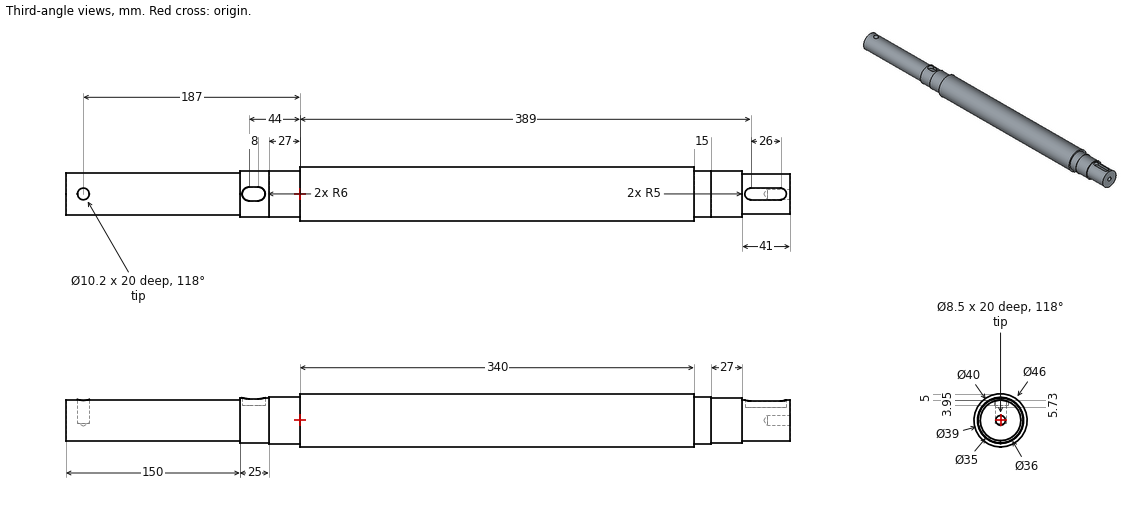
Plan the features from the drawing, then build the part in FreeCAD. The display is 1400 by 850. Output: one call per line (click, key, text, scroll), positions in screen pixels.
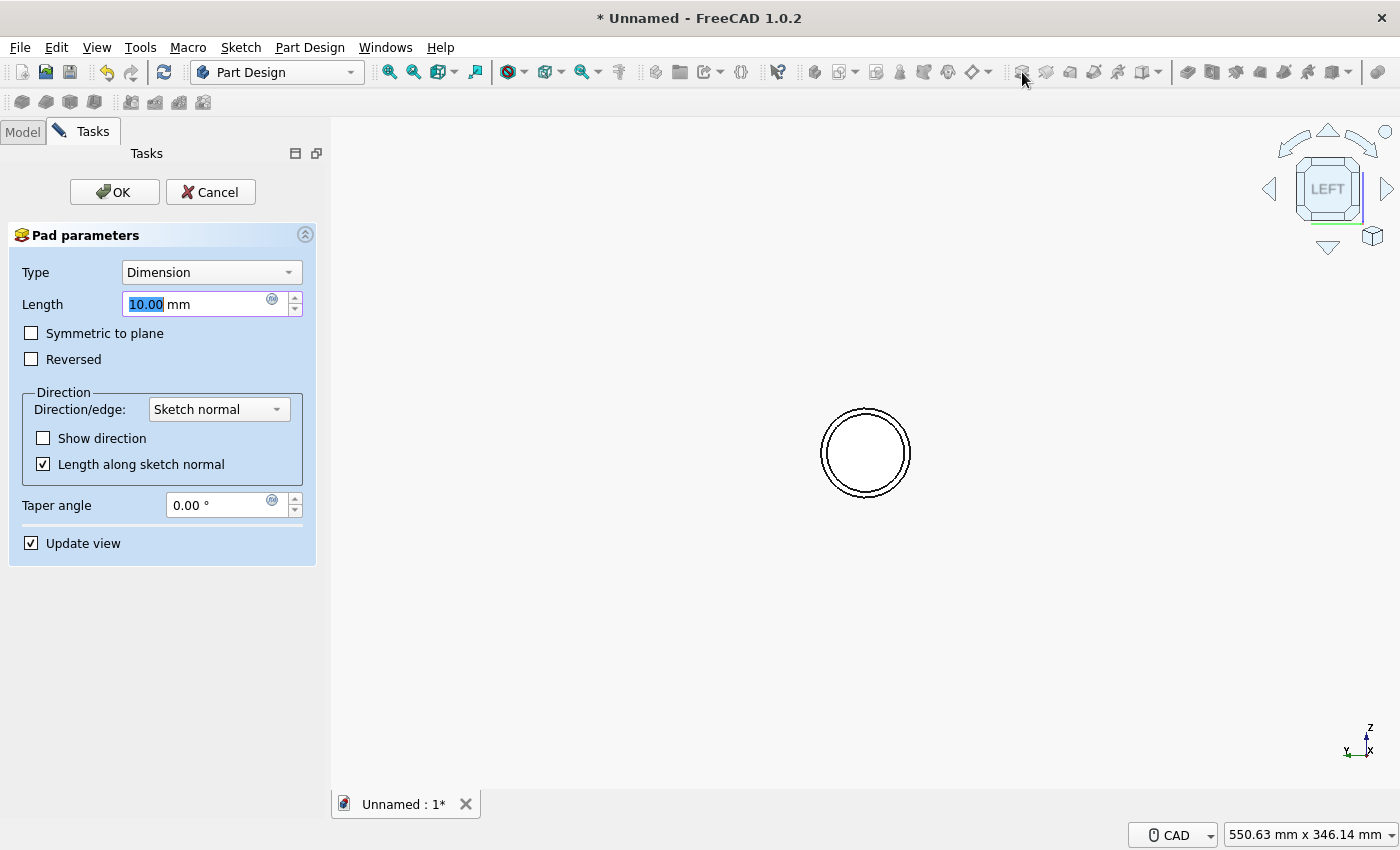
text(27)
key(Tab)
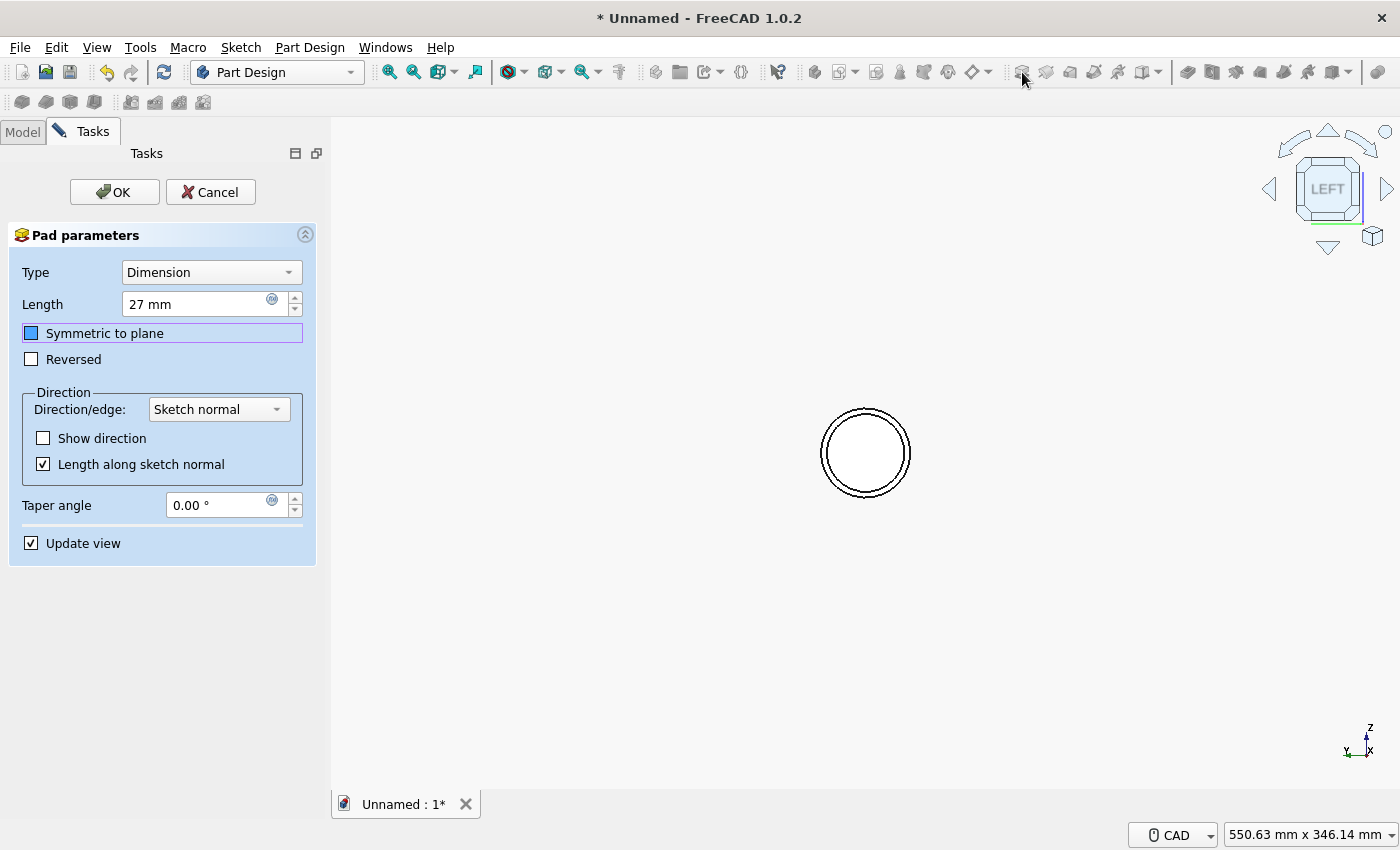
click(115, 192)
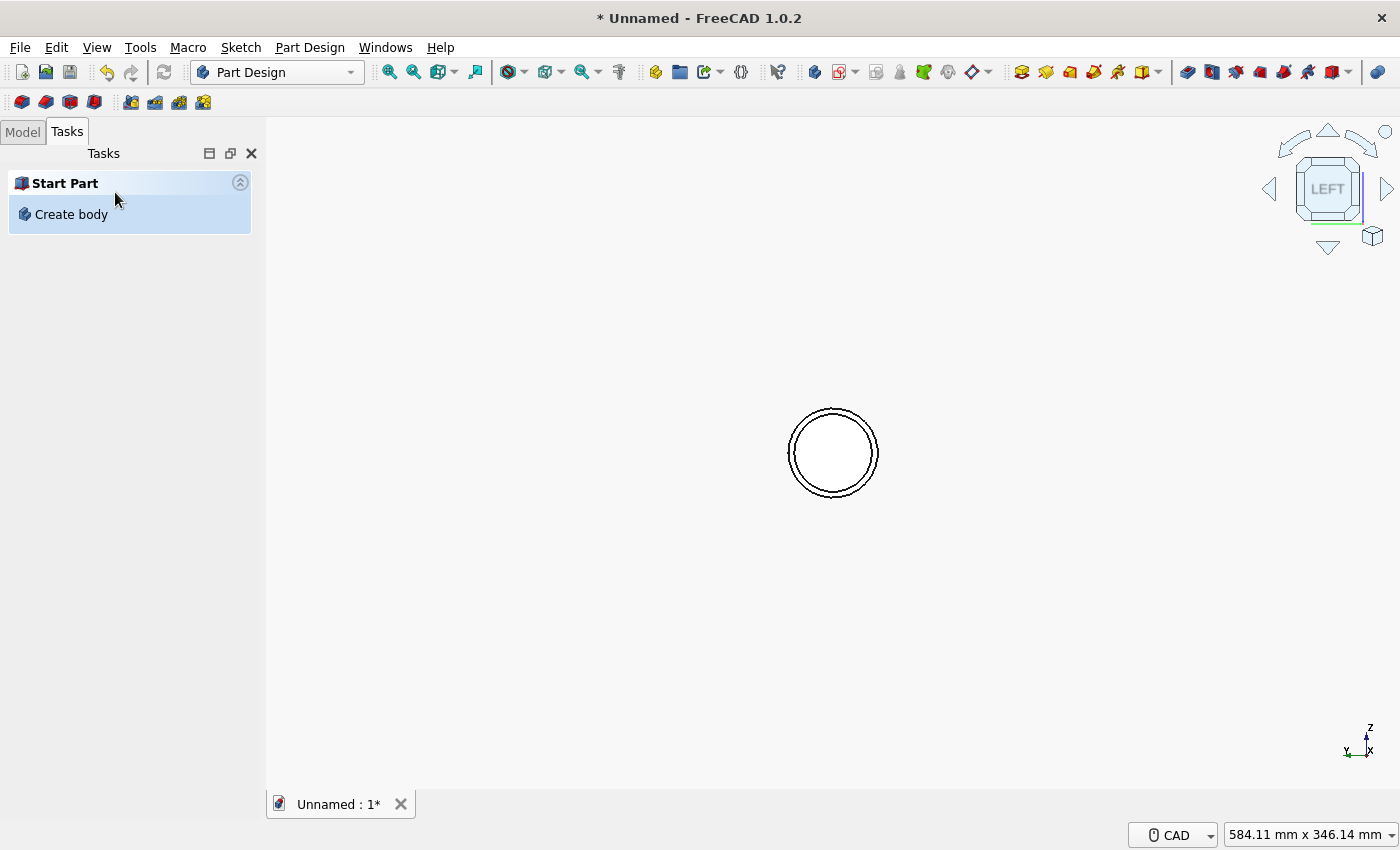
click(390, 72)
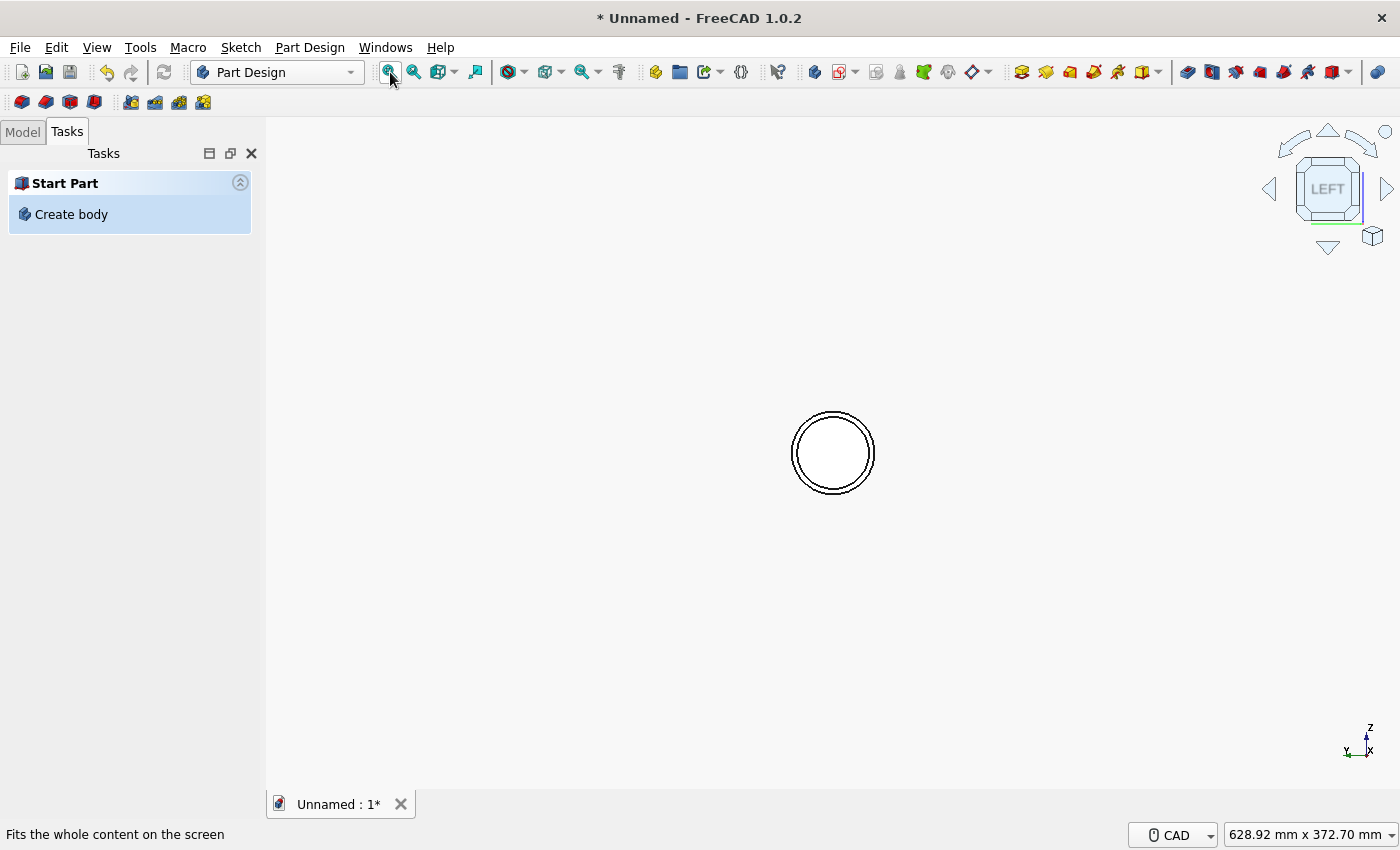
click(833, 452)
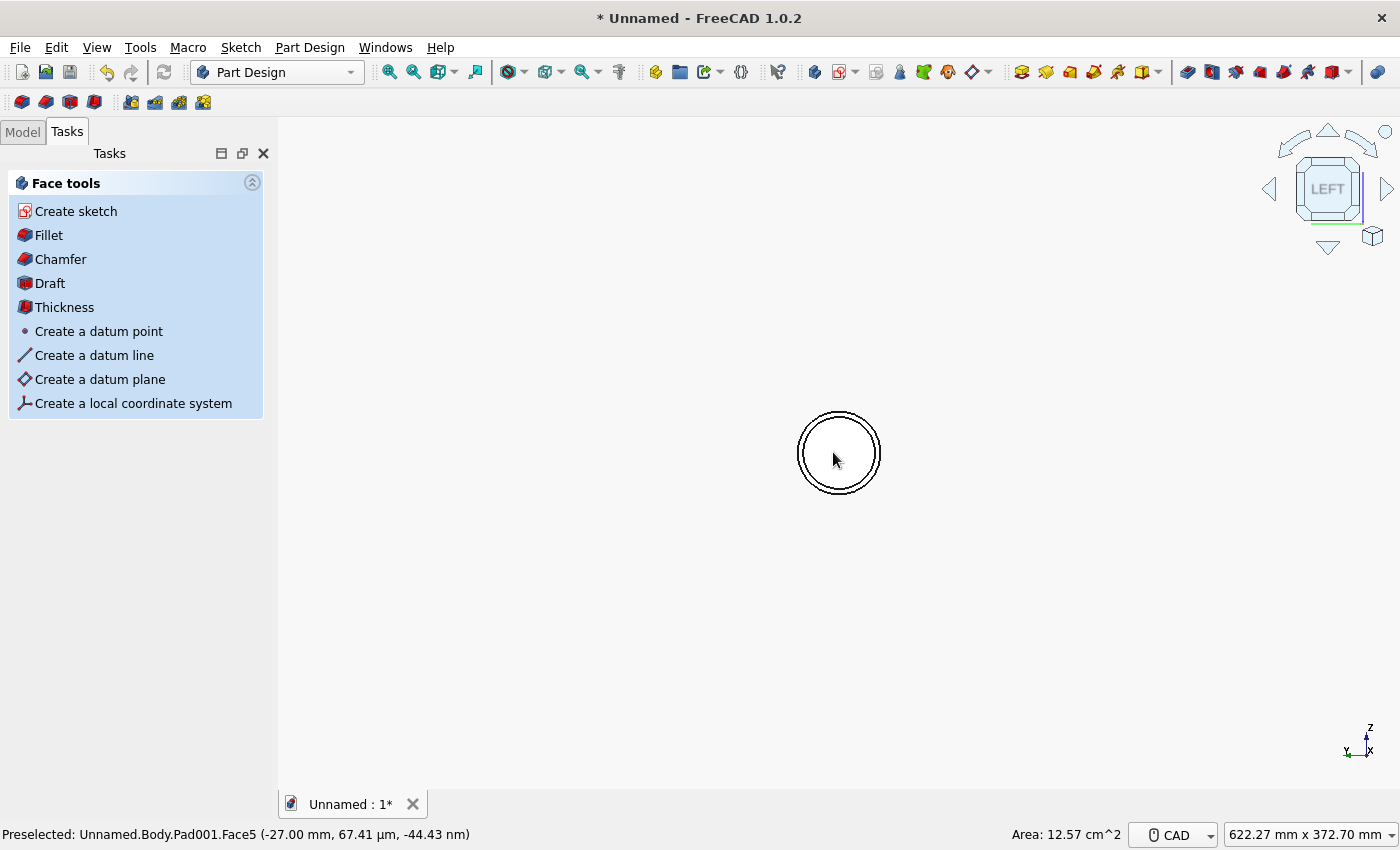
click(840, 72)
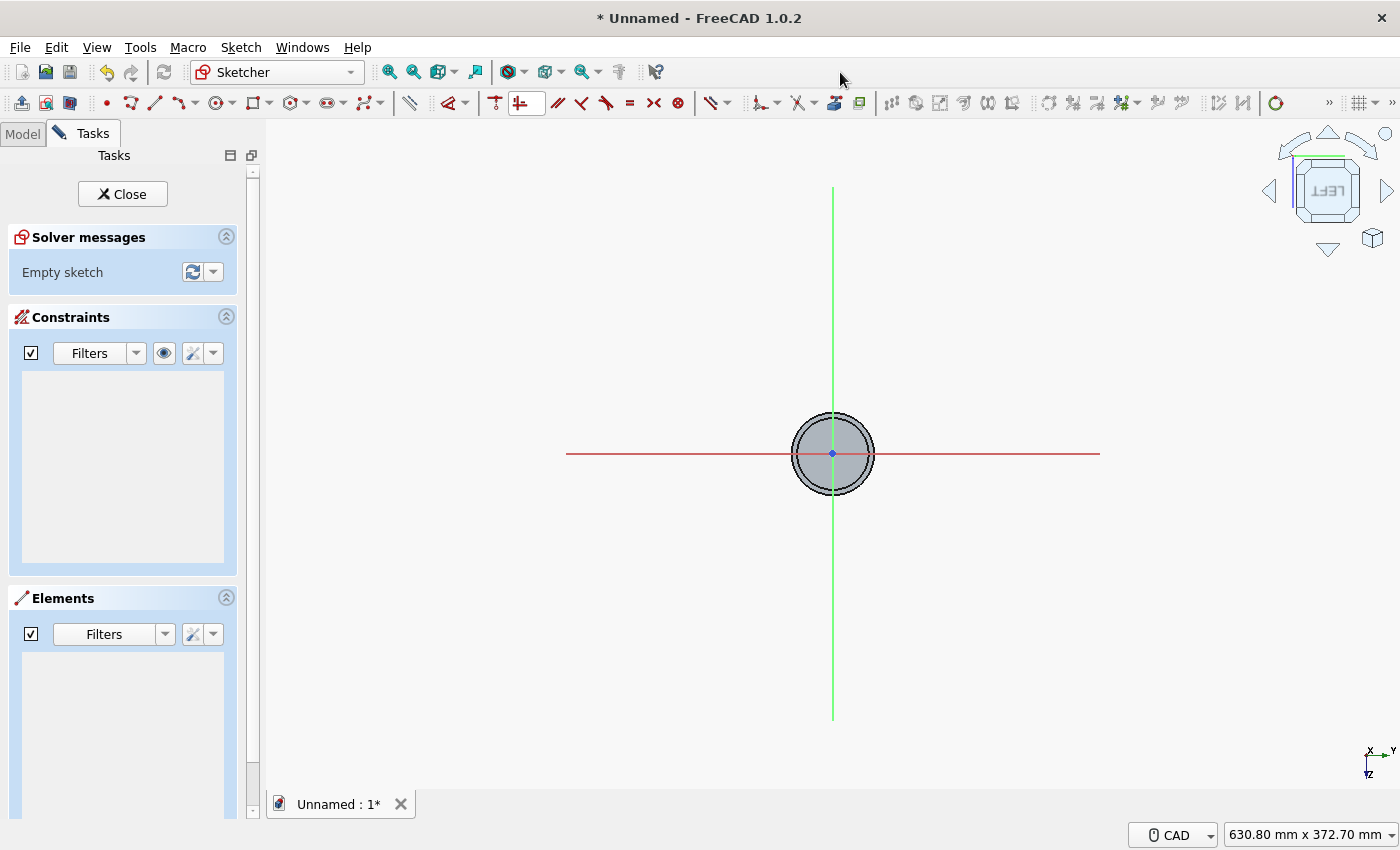
scroll(846, 454, up, 9)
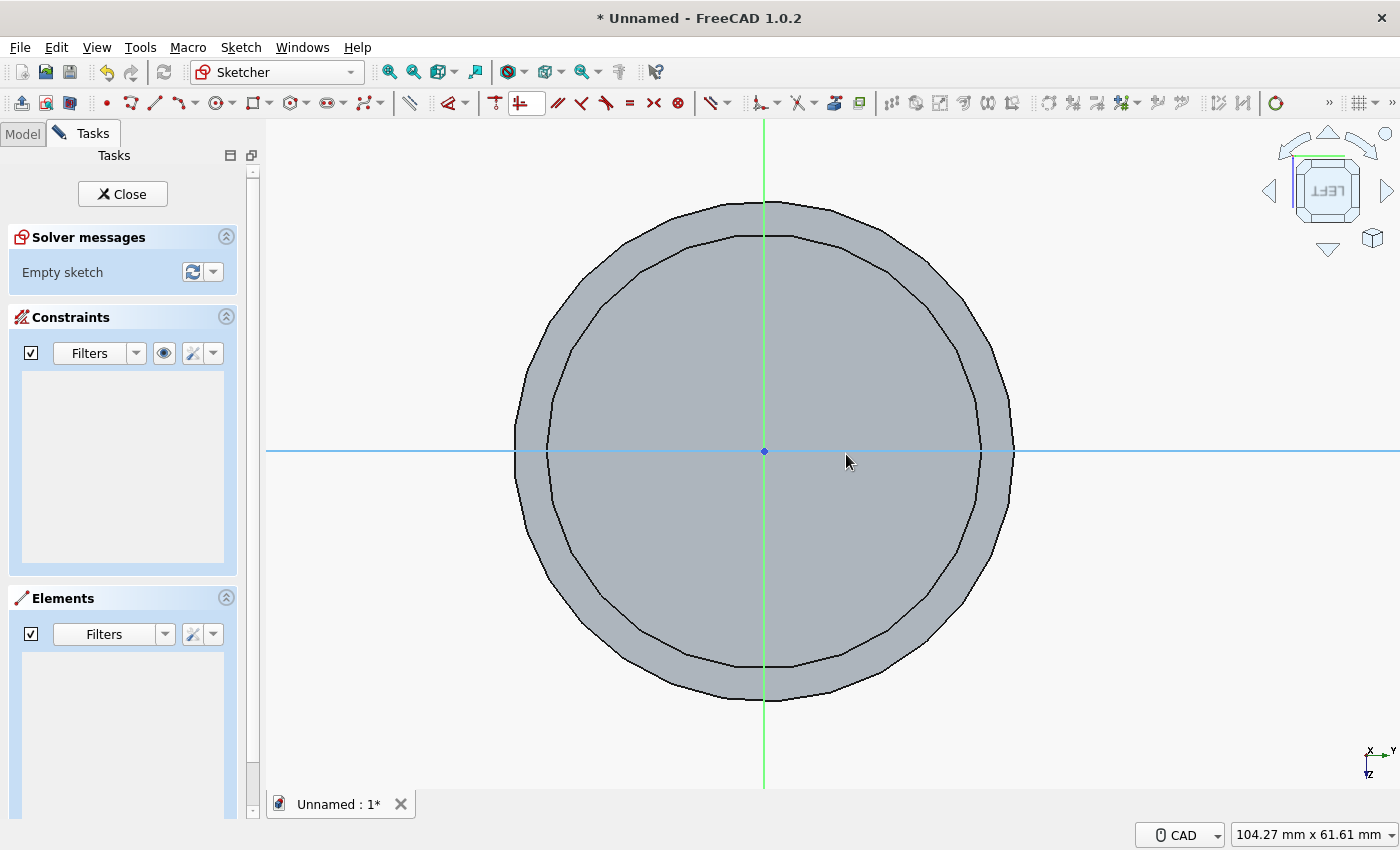
click(216, 104)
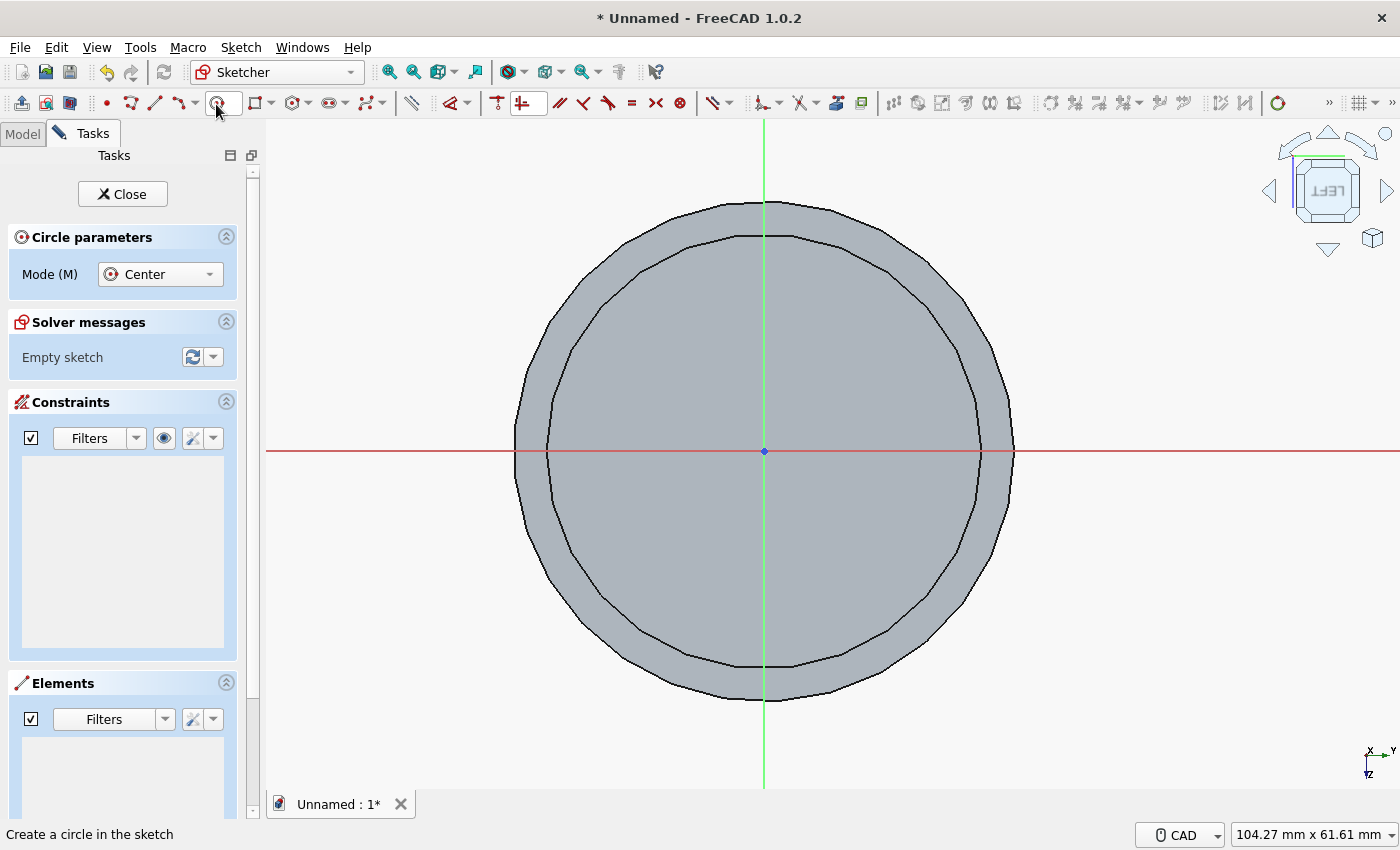
click(764, 451)
click(914, 302)
key(Escape)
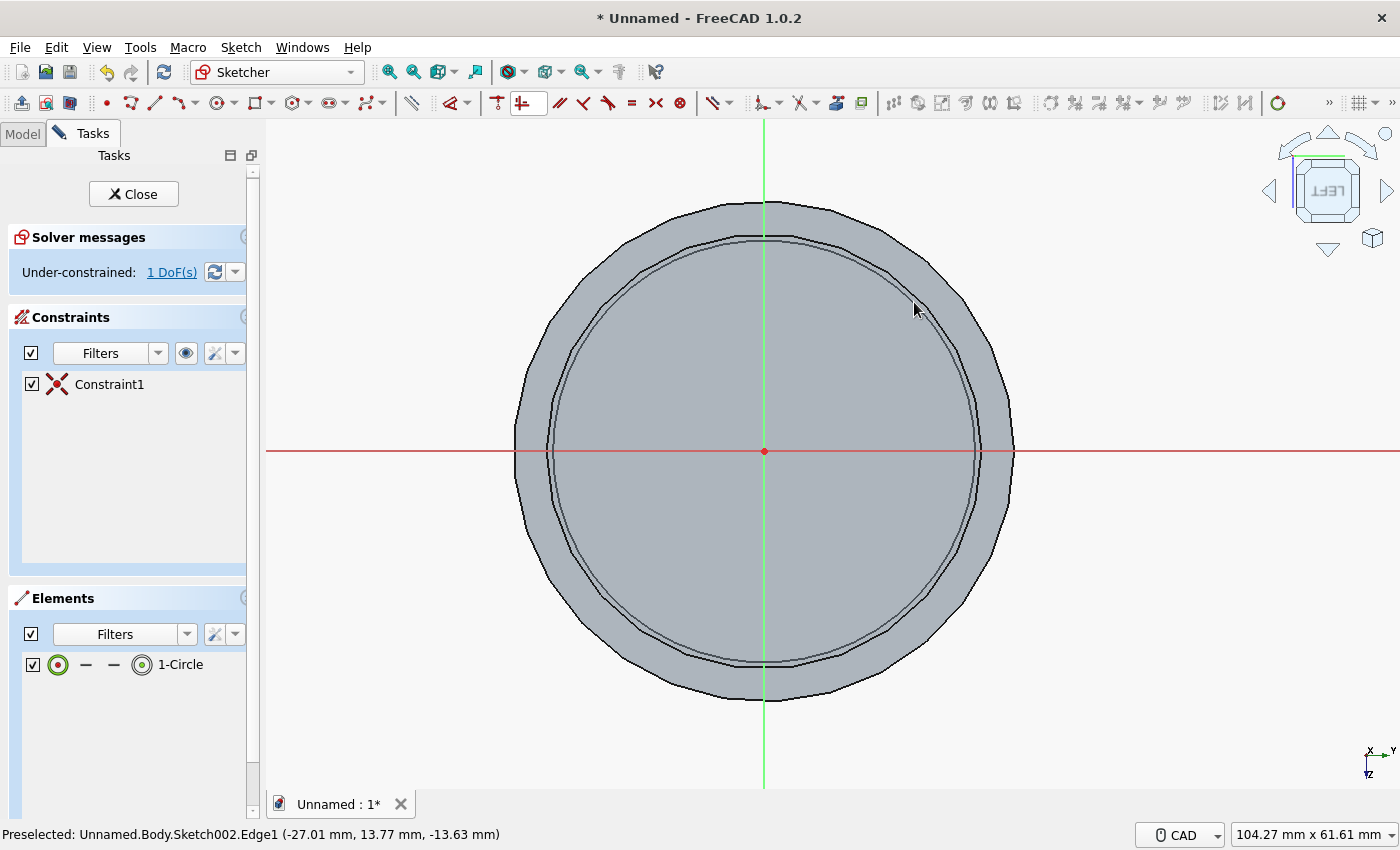
click(450, 104)